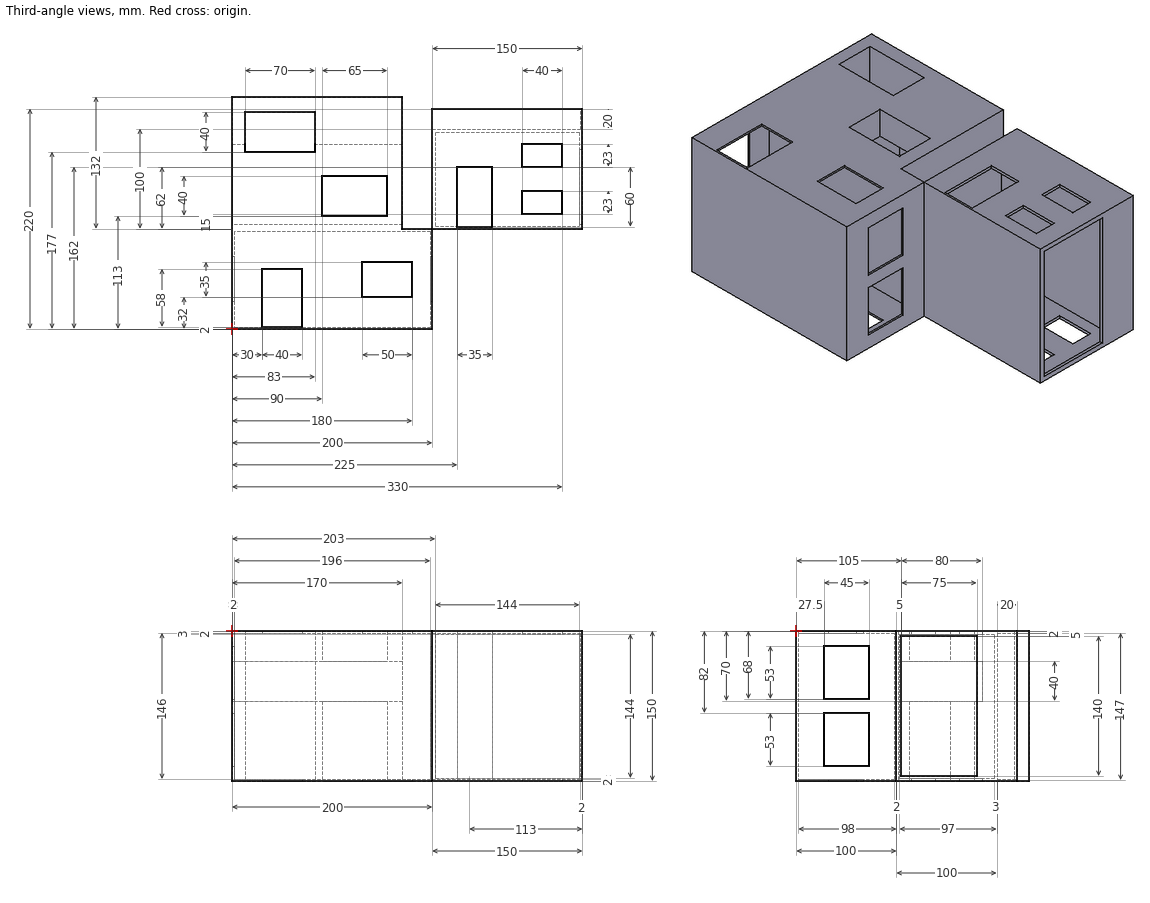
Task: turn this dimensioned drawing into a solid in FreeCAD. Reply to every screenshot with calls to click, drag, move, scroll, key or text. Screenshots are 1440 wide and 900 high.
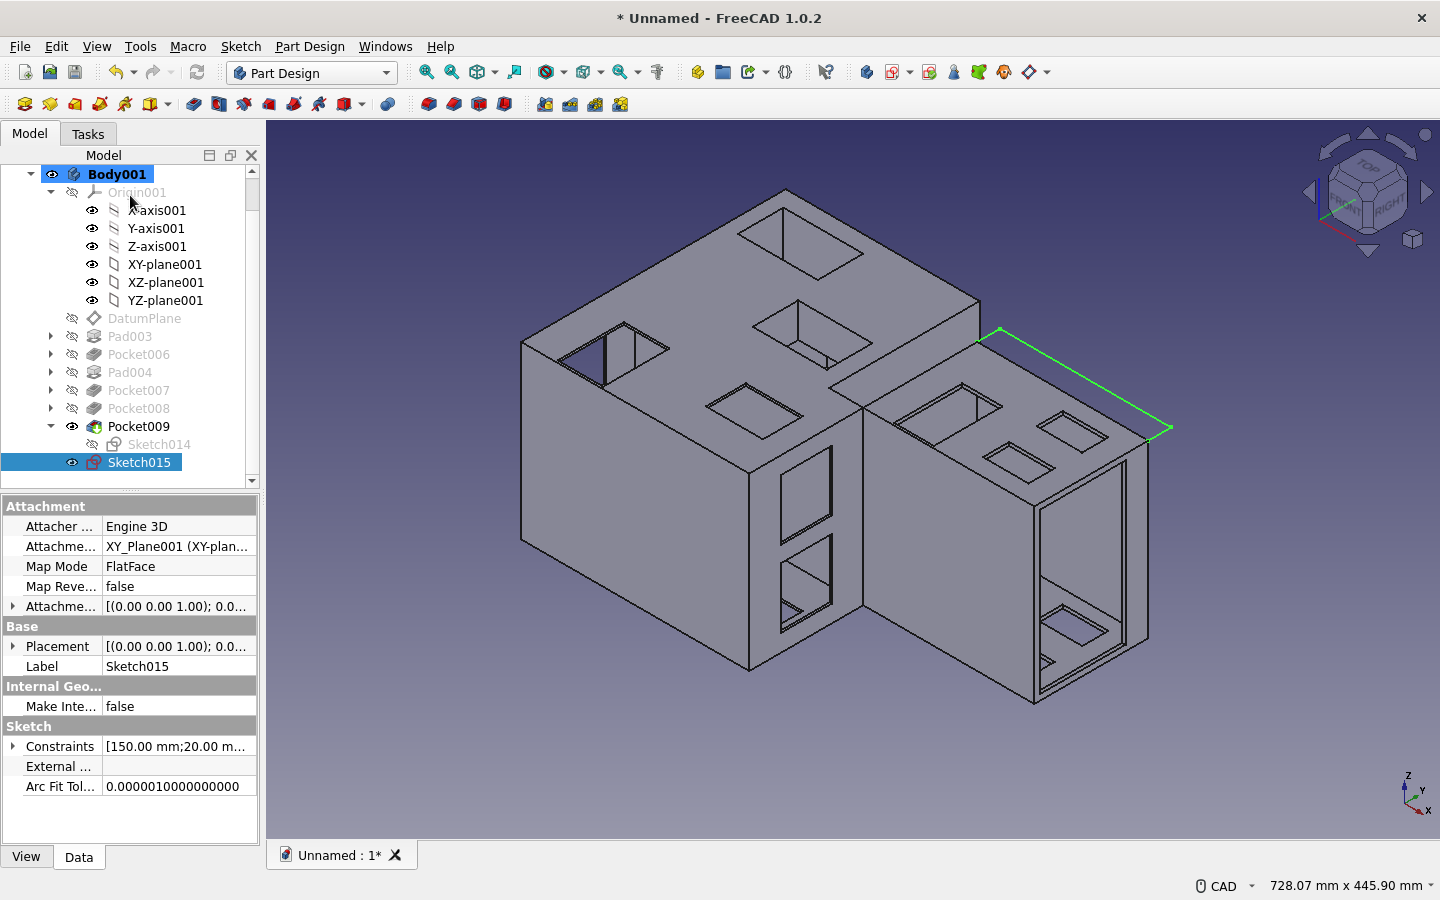
click(25, 104)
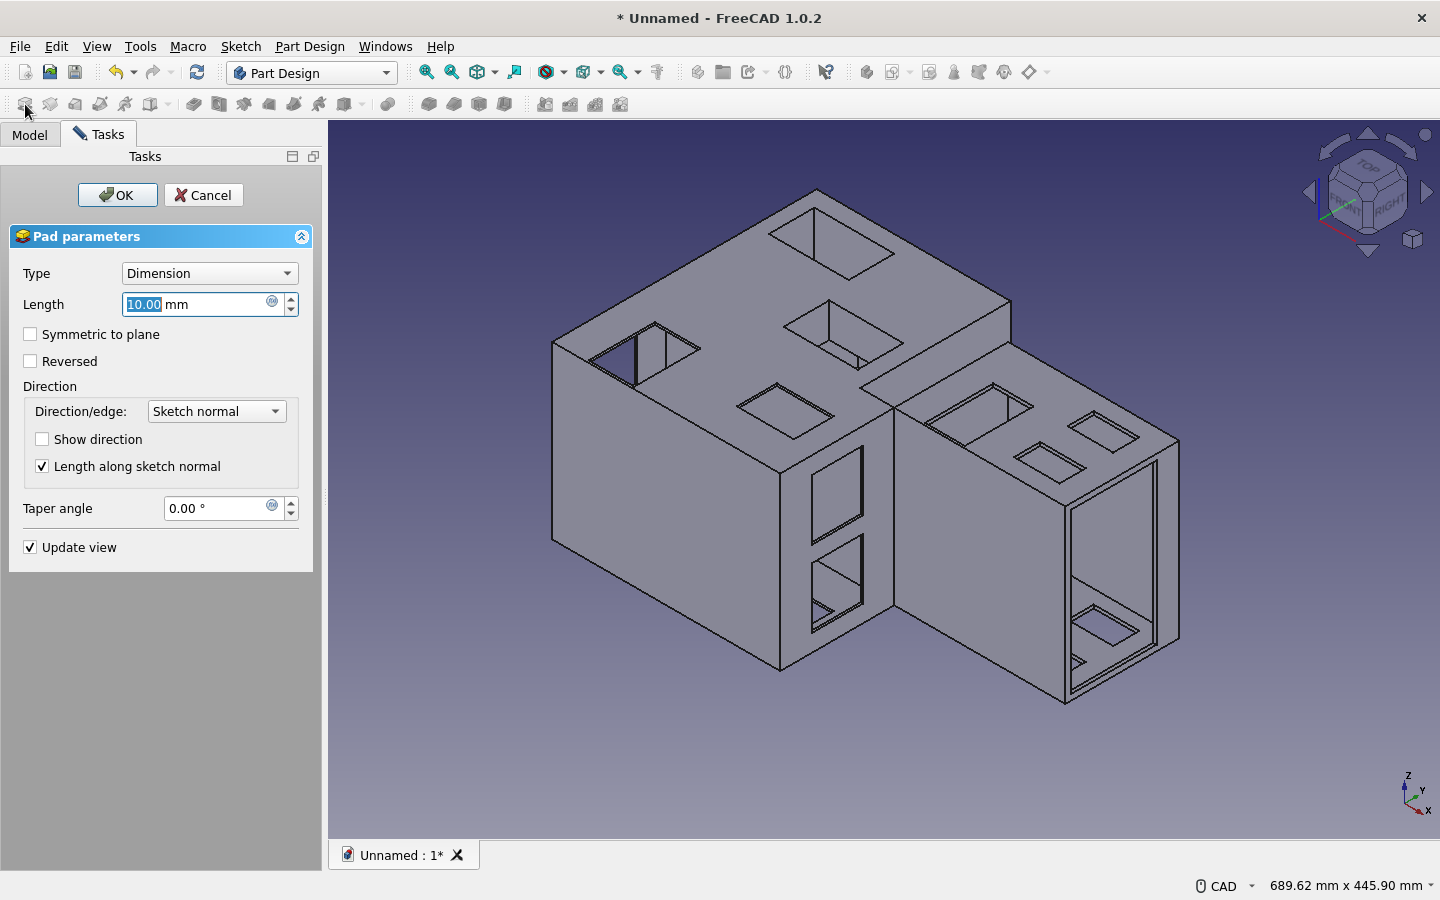
text(2)
key(Tab)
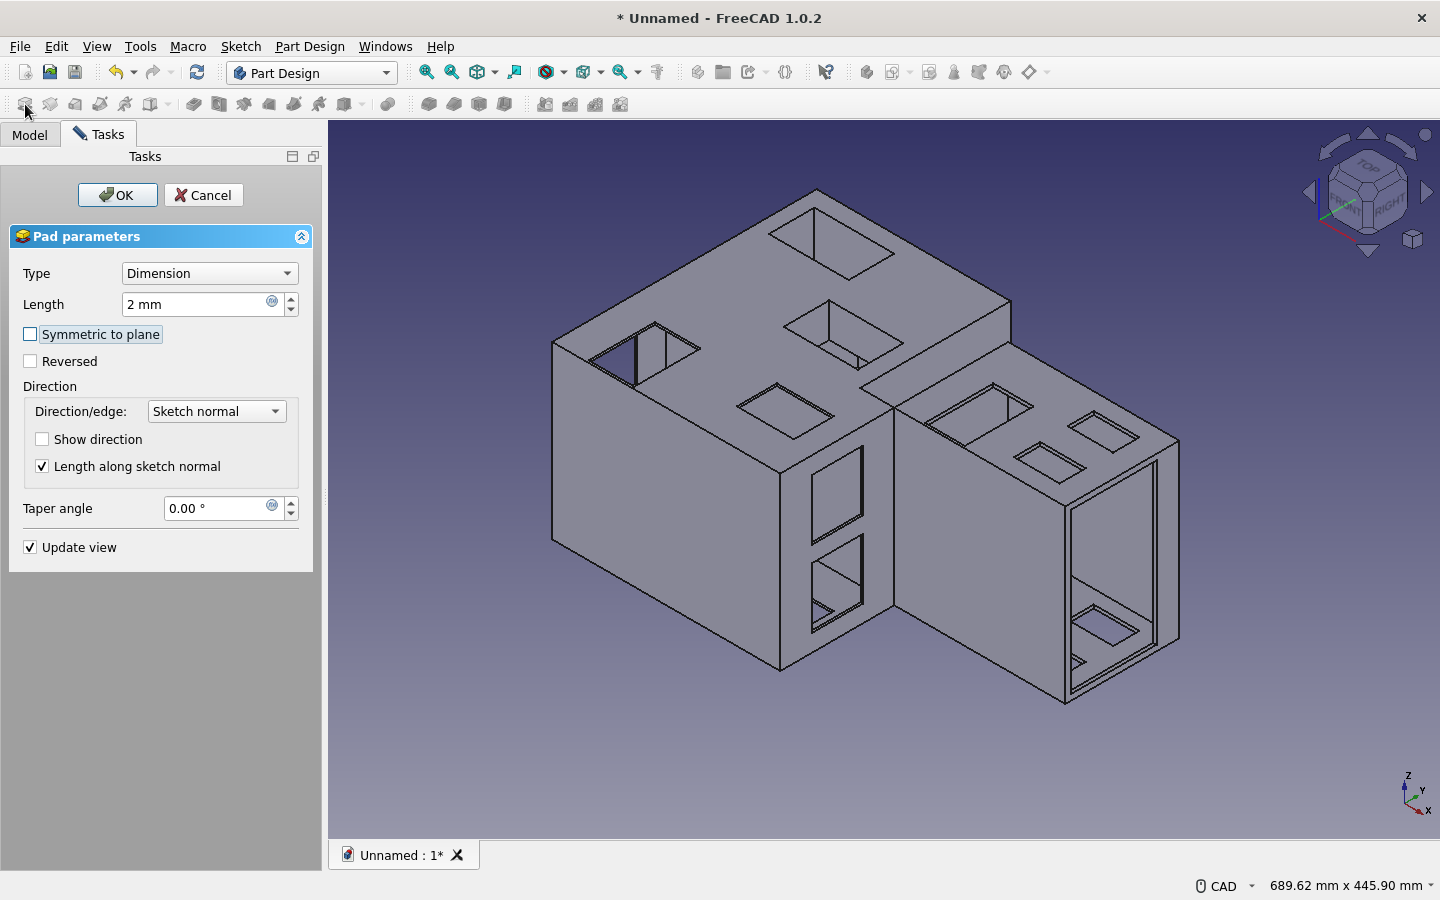
click(31, 361)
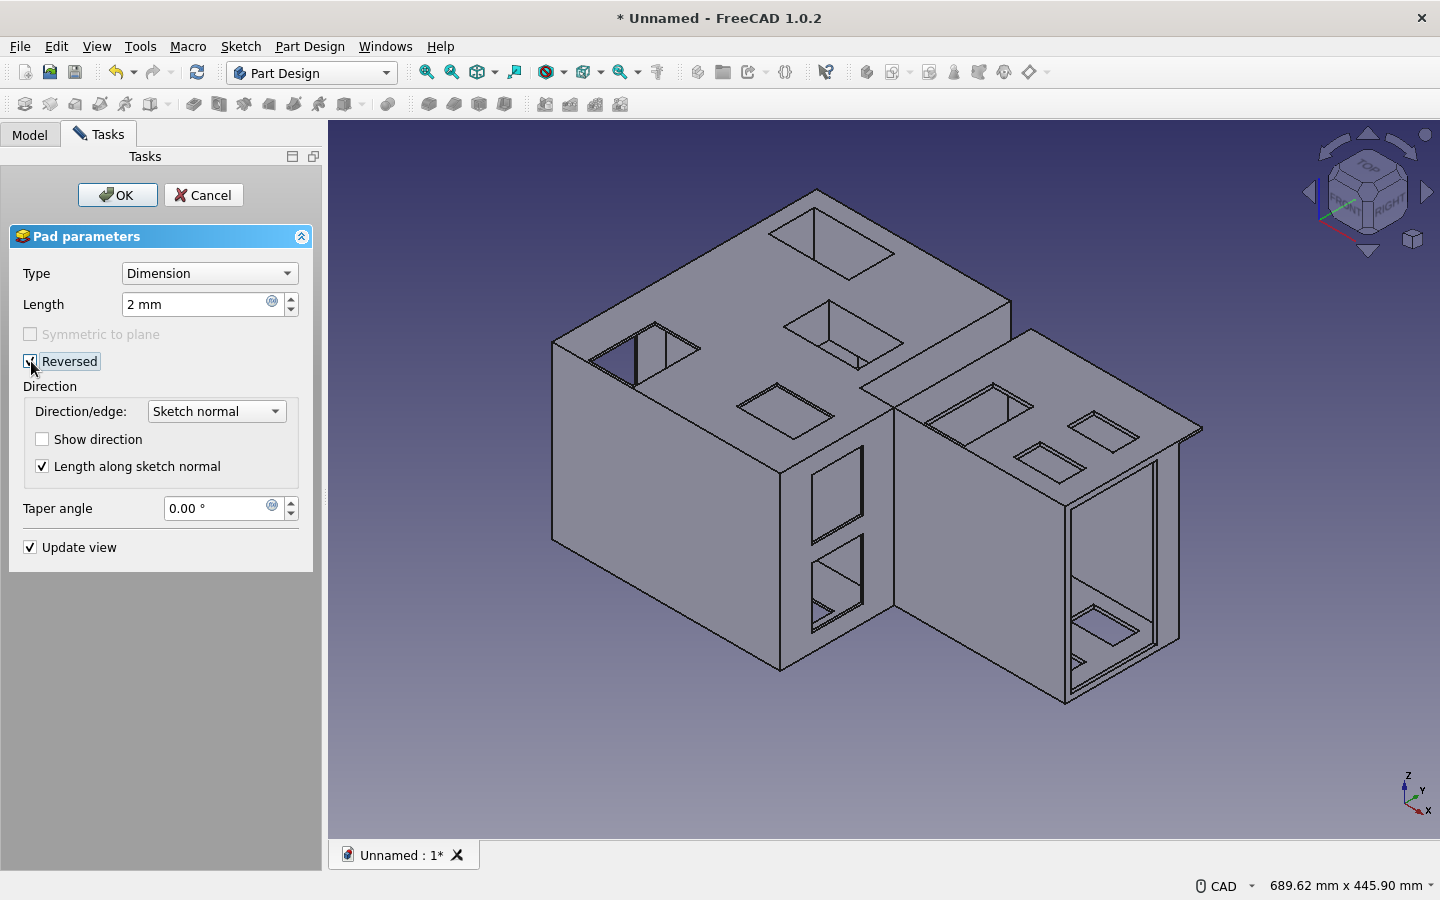
click(118, 195)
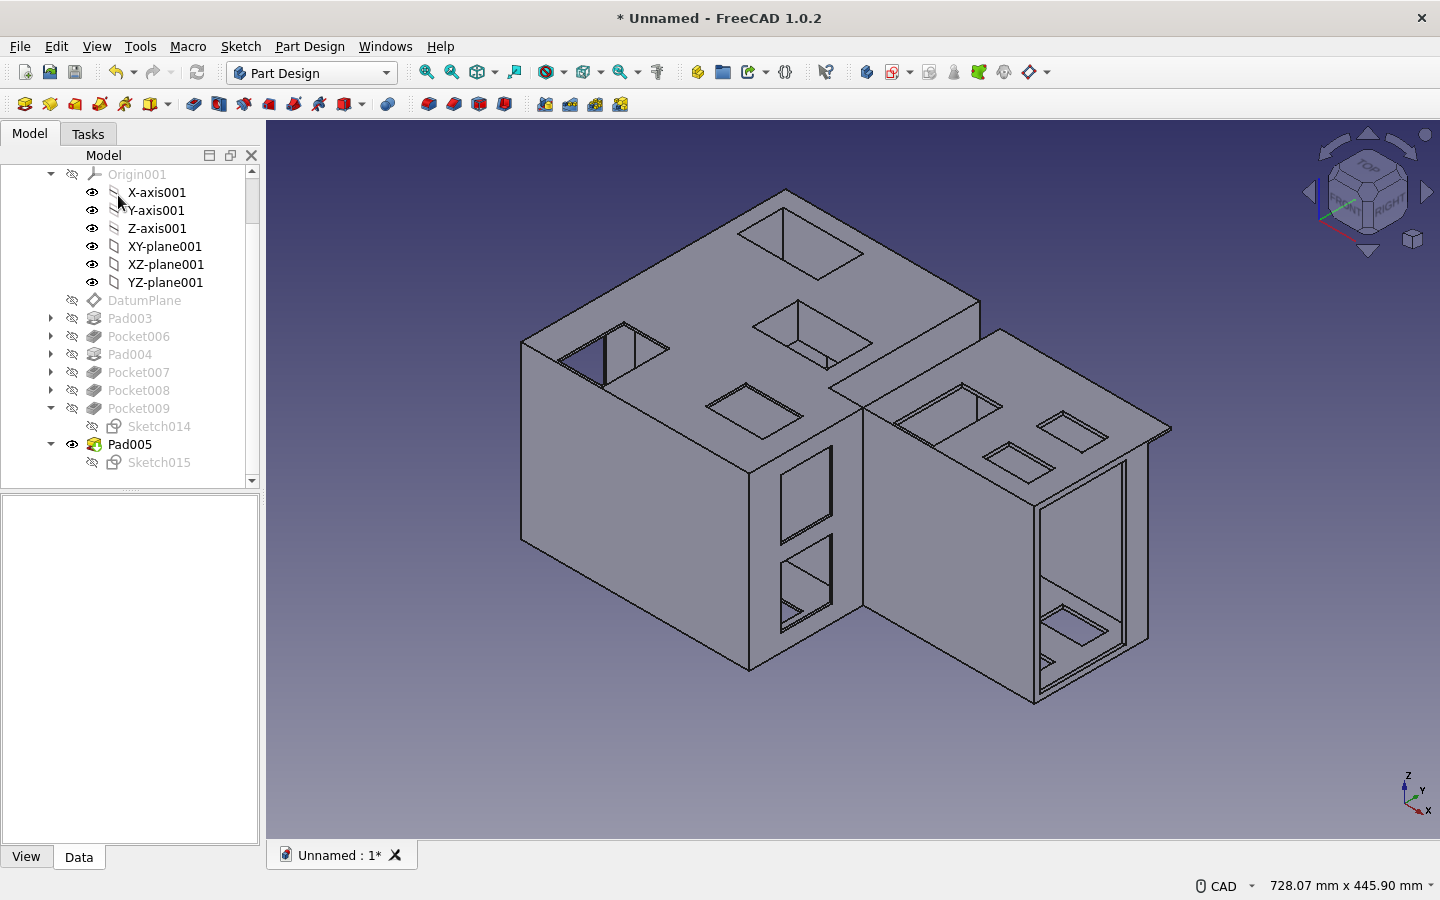
click(1142, 458)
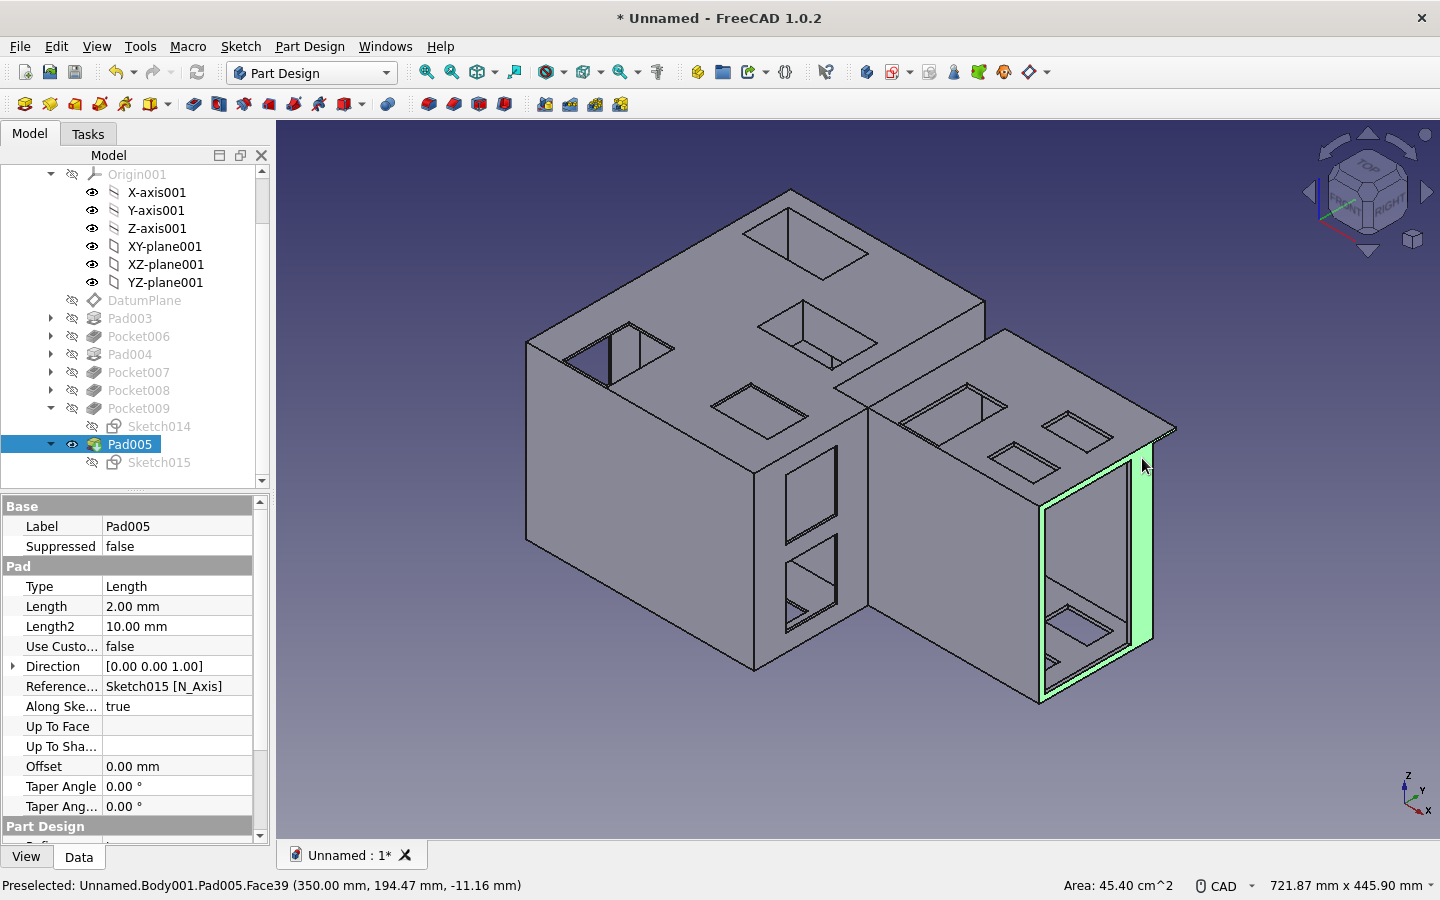
click(892, 72)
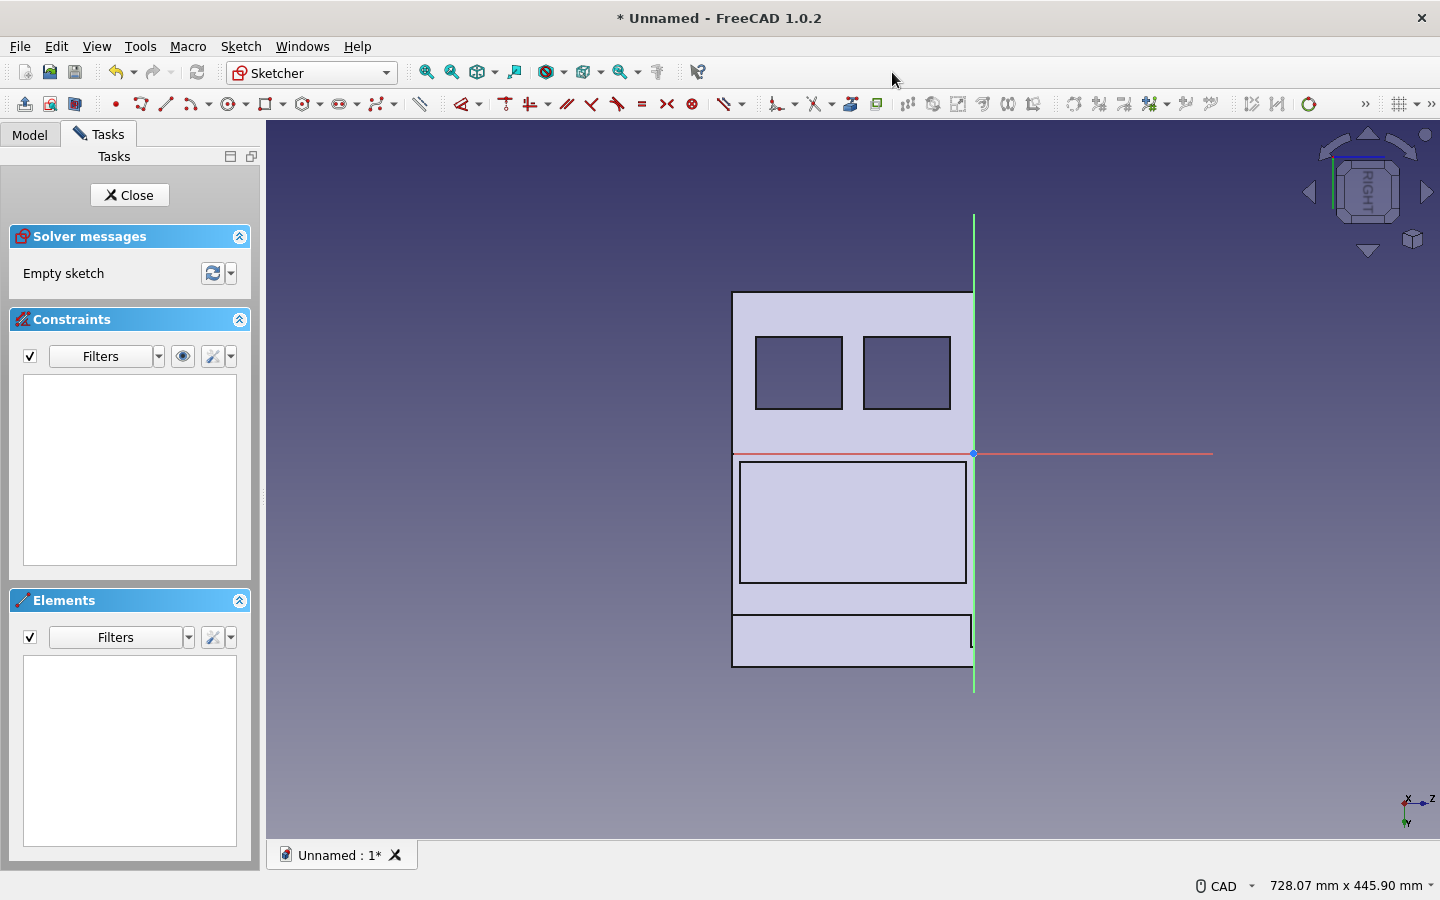
scroll(910, 608, up, 4)